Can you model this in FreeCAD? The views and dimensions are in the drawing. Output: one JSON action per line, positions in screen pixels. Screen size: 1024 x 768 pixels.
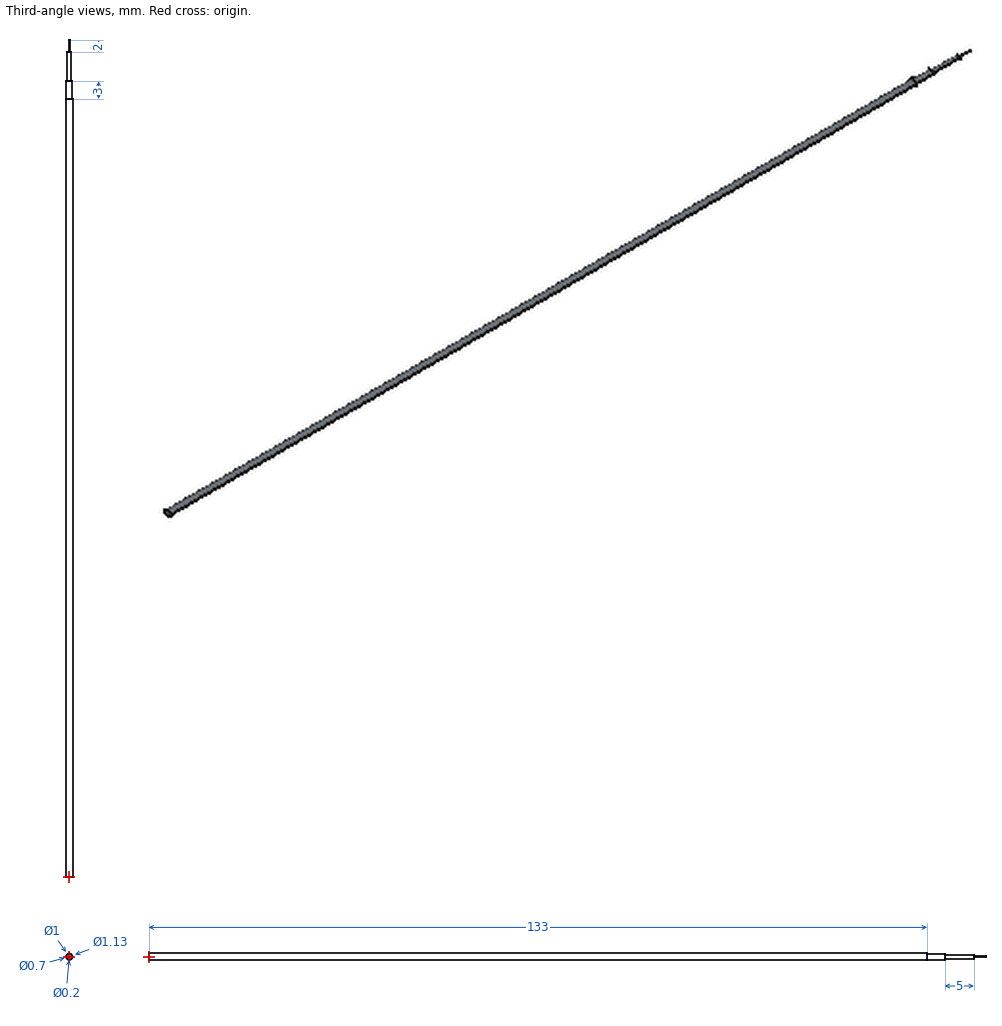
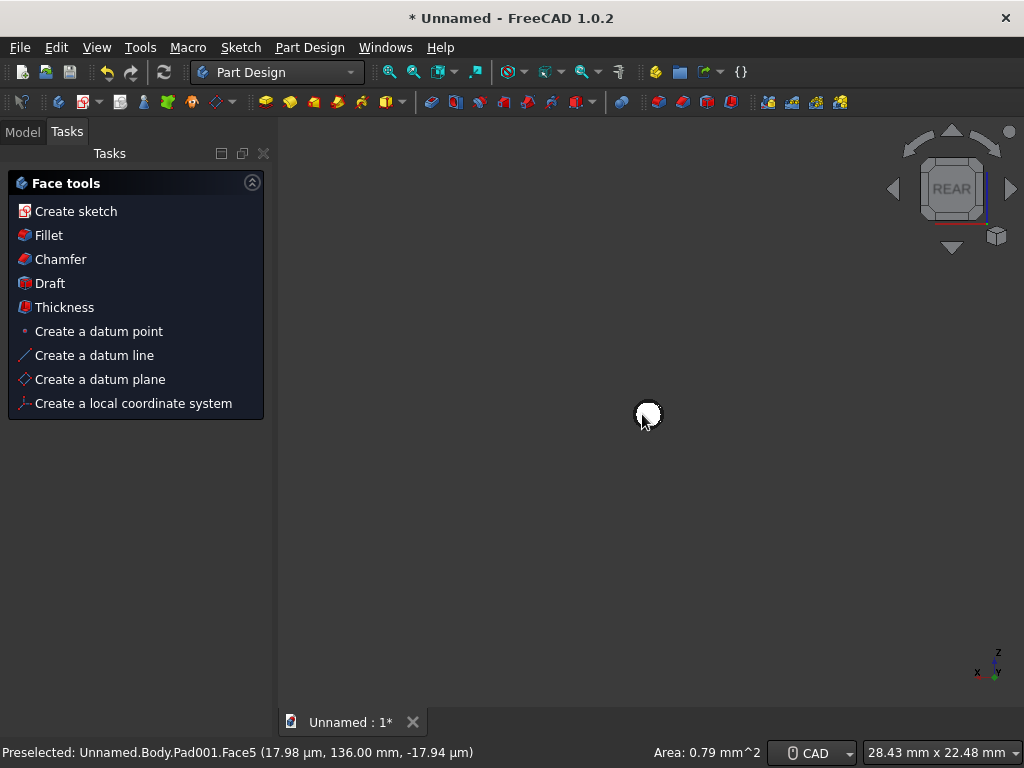
{"action": "left_click", "coordinate": [84, 102]}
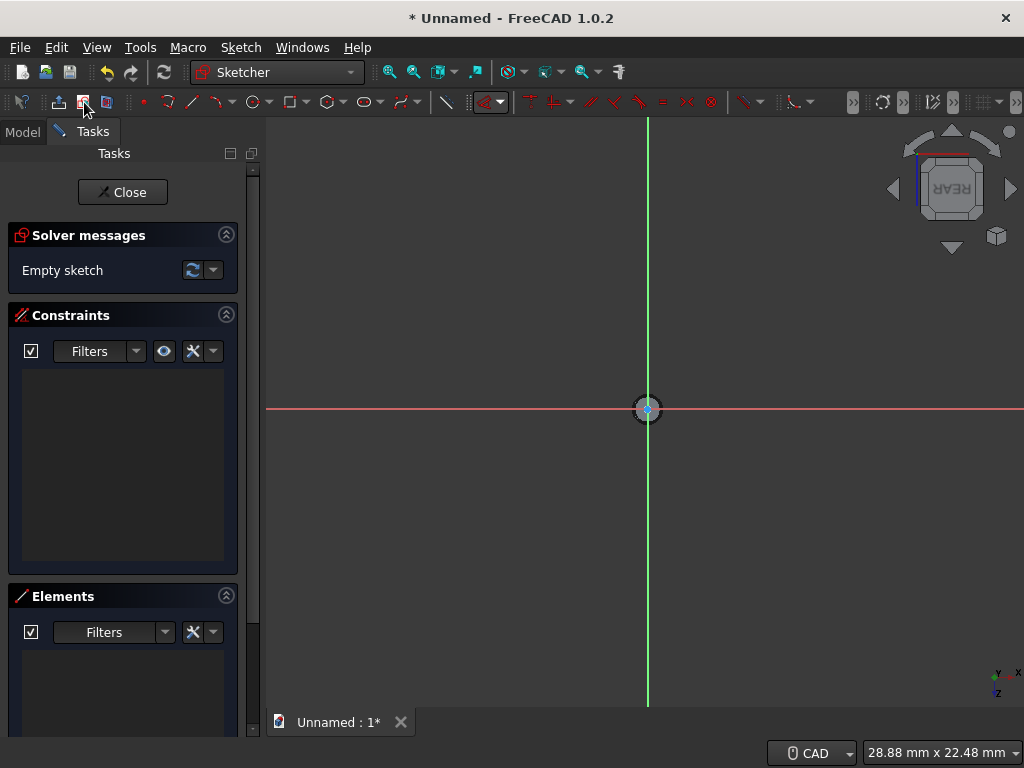
{"action": "scroll", "coordinate": [651, 409], "scroll_direction": "up", "scroll_amount": 15}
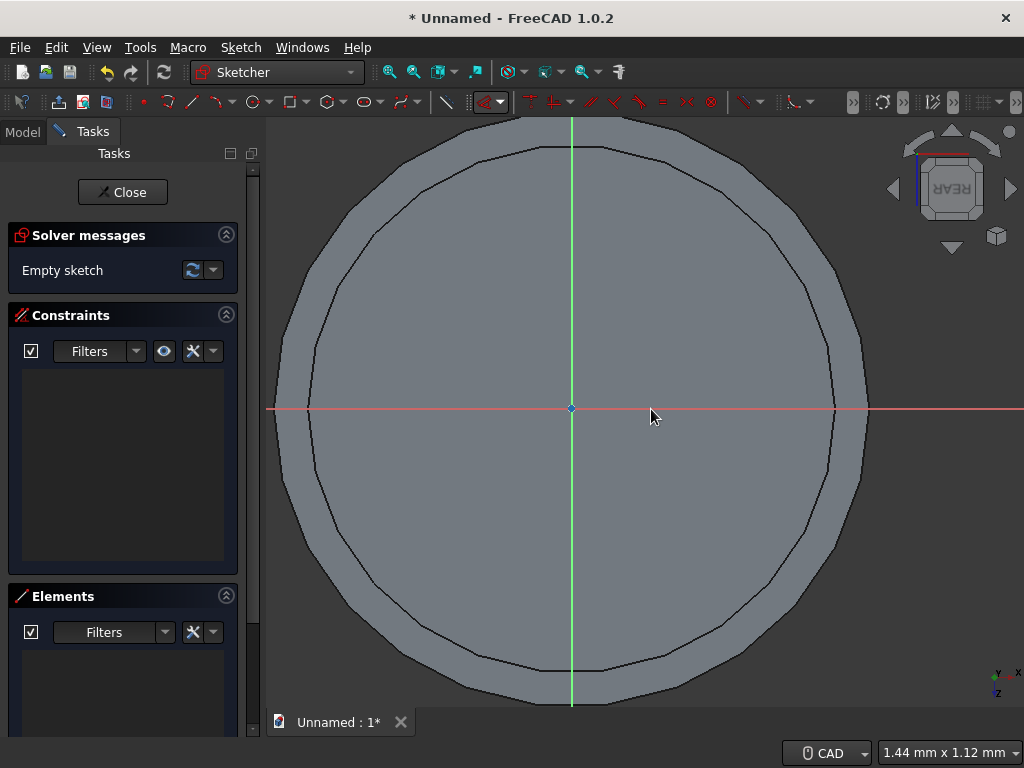
{"action": "left_click", "coordinate": [254, 102]}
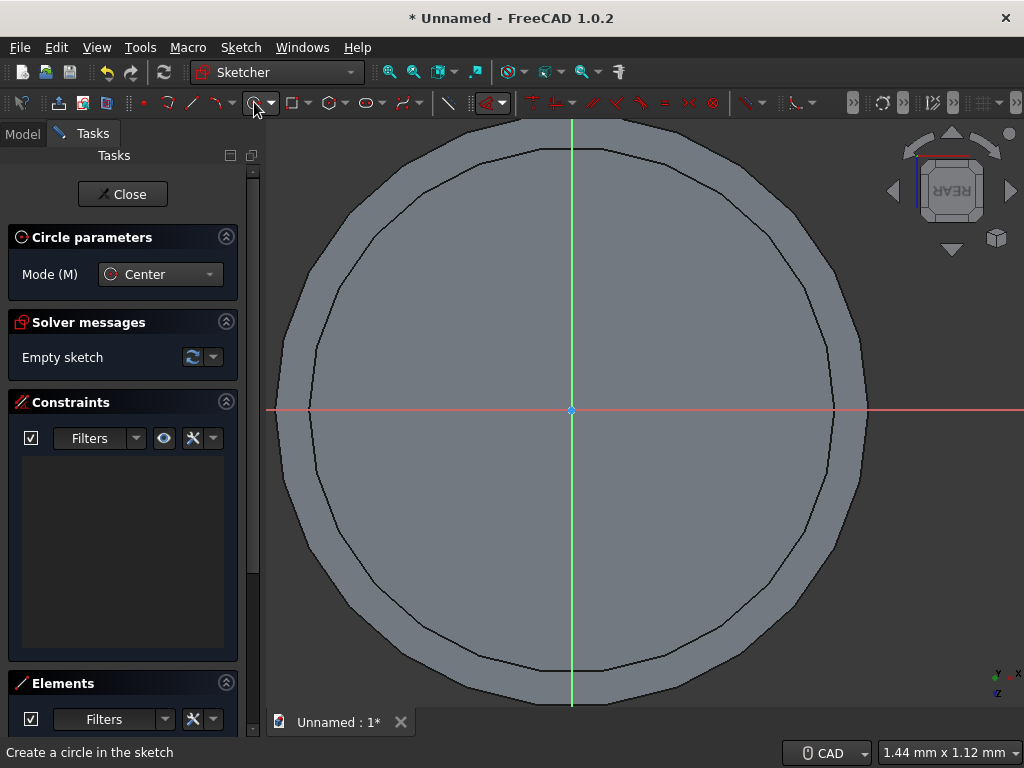
{"action": "left_click", "coordinate": [572, 410]}
{"action": "left_click", "coordinate": [702, 280]}
{"action": "key", "text": "Escape"}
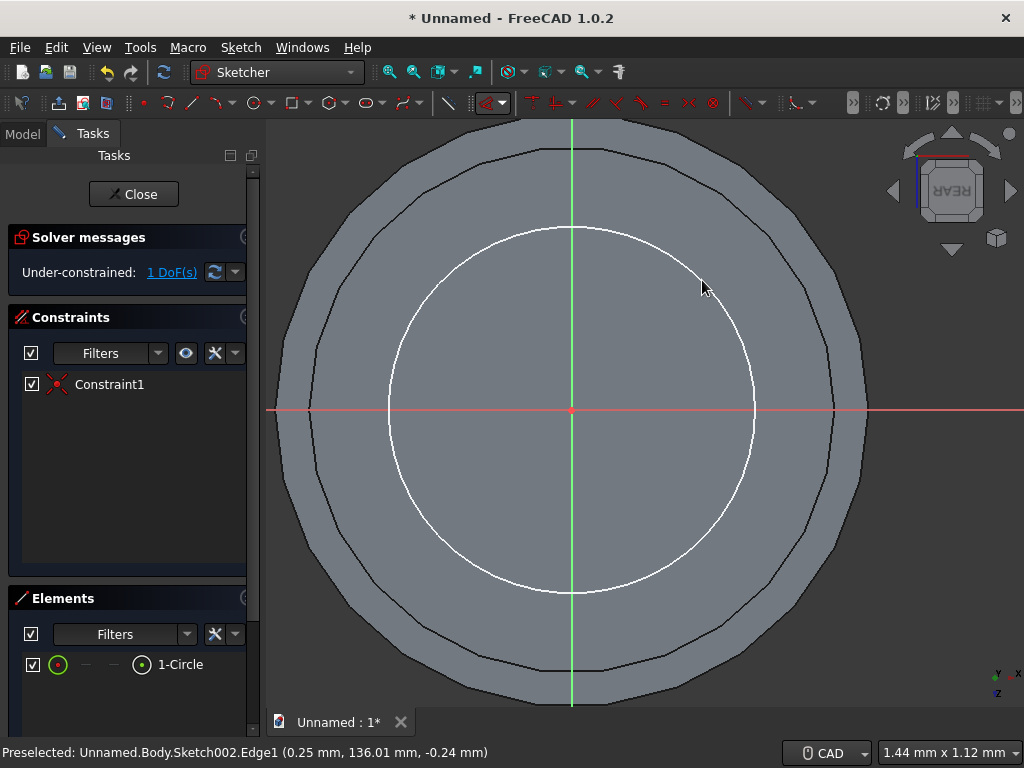
{"action": "left_click", "coordinate": [701, 280]}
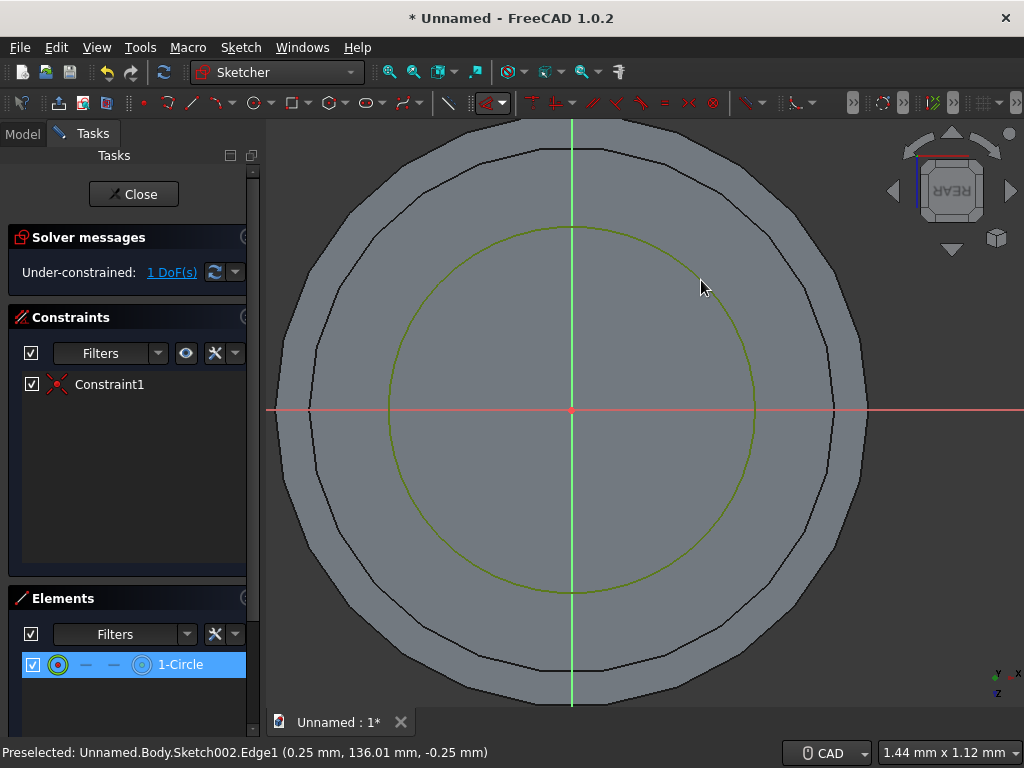
{"action": "left_click", "coordinate": [504, 104]}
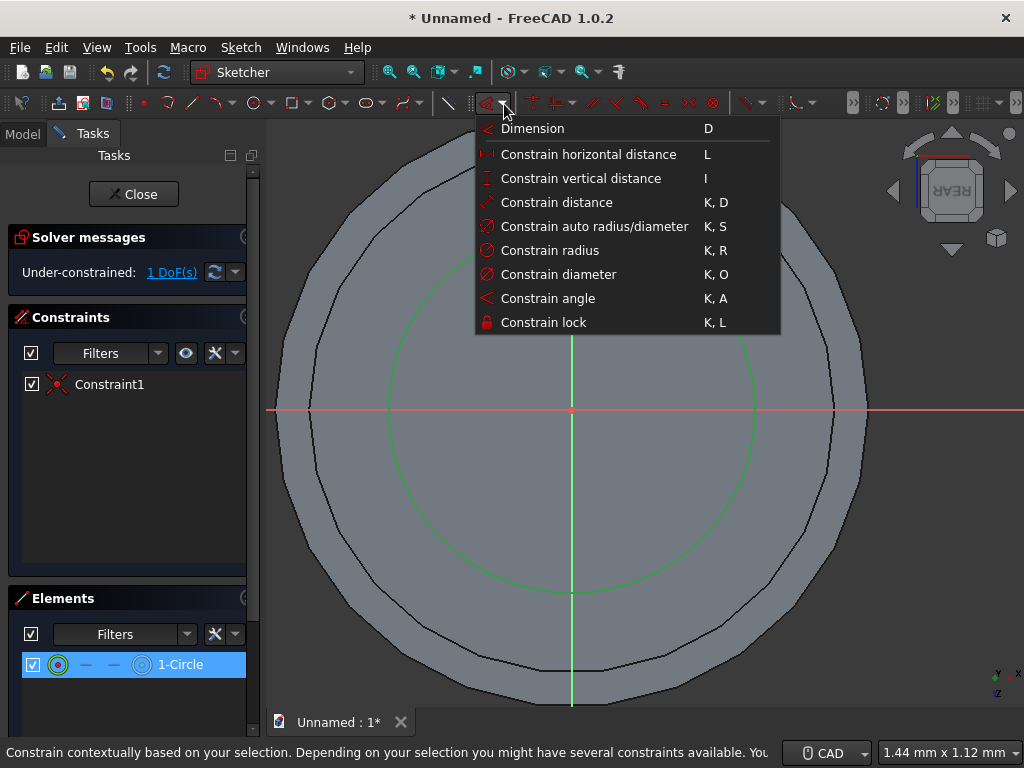
{"action": "left_click", "coordinate": [628, 274]}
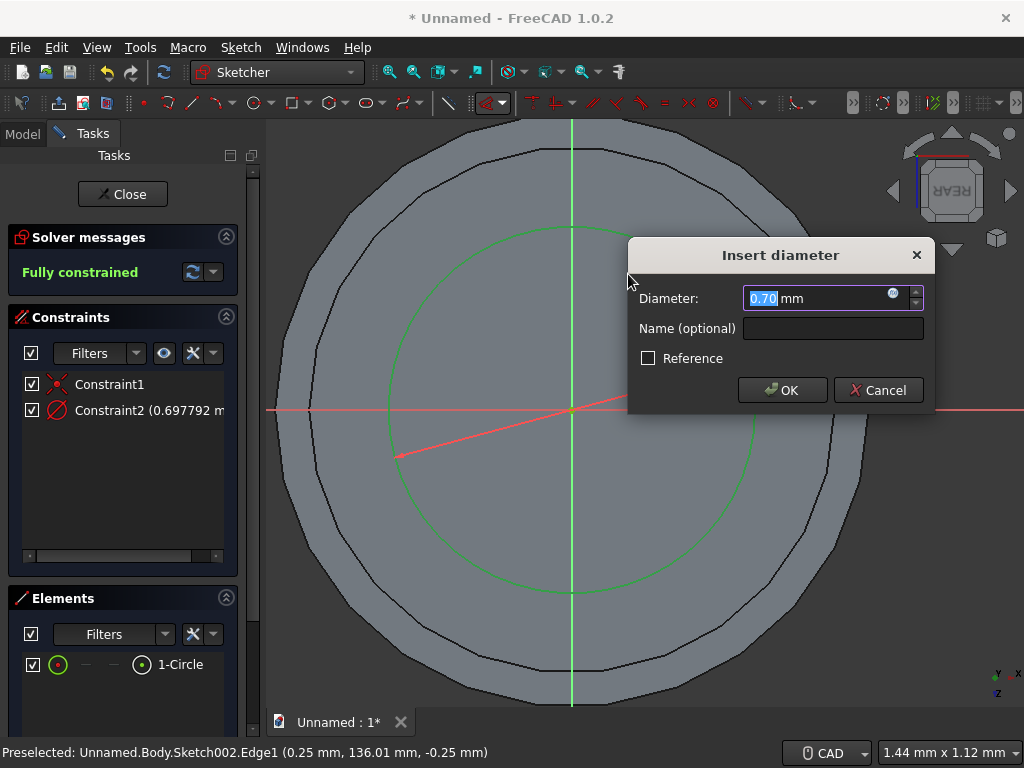
{"action": "type", "text": "0.7"}
{"action": "key", "text": "Return"}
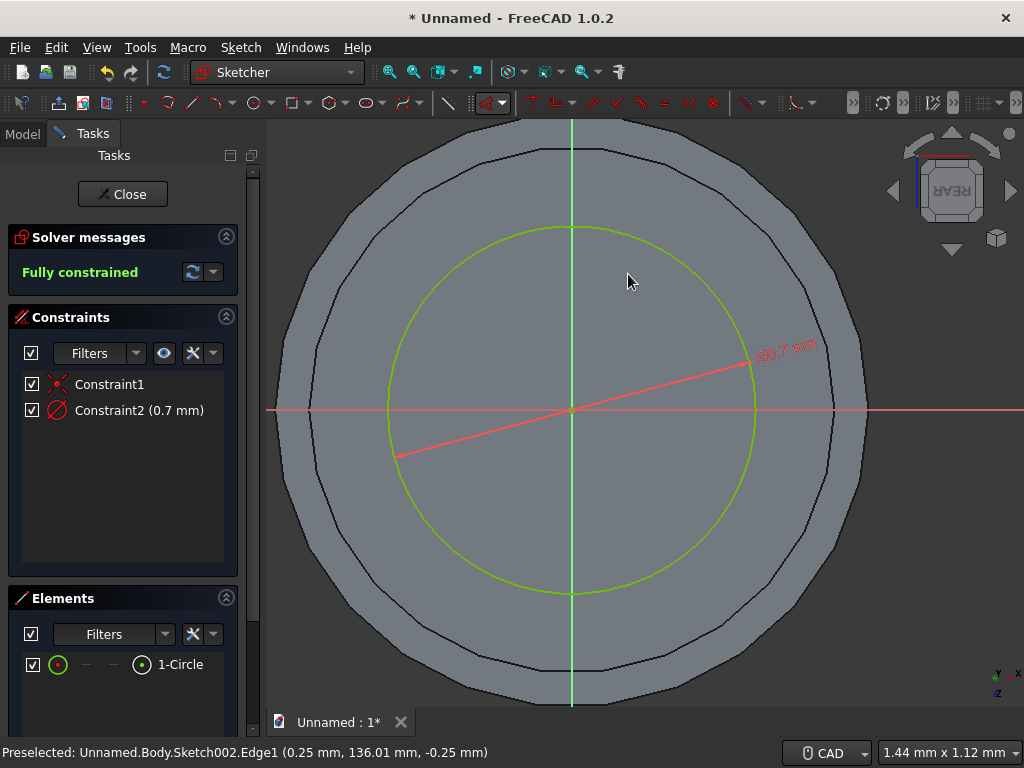
{"action": "left_click", "coordinate": [123, 194]}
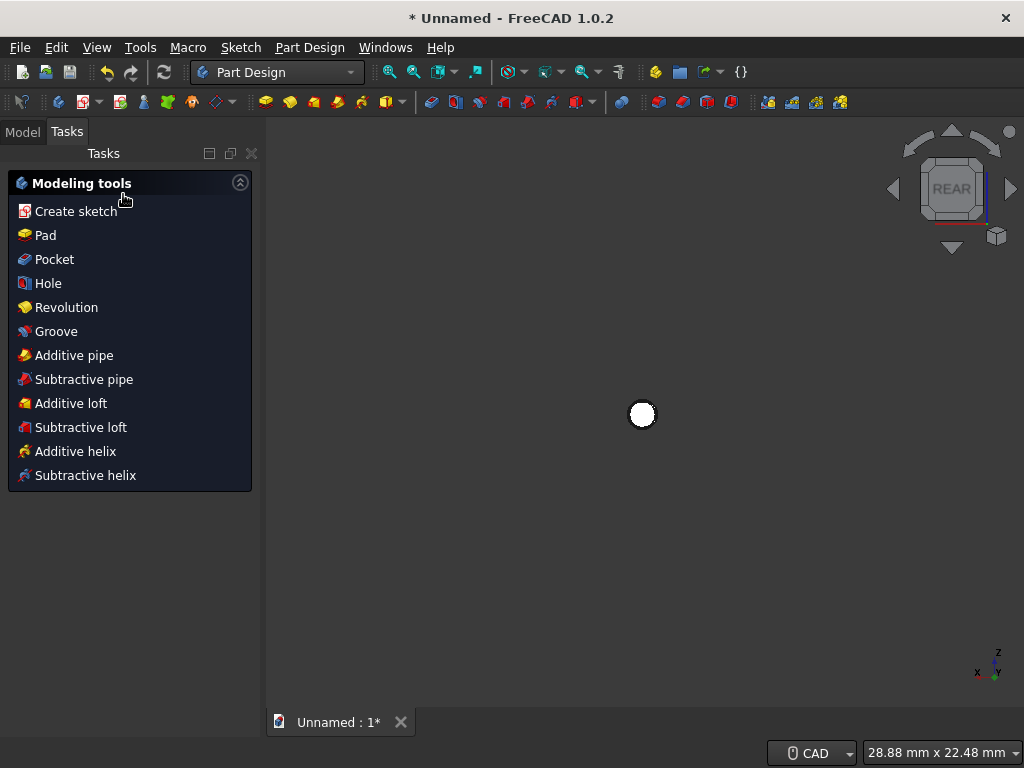
{"action": "left_click", "coordinate": [266, 102]}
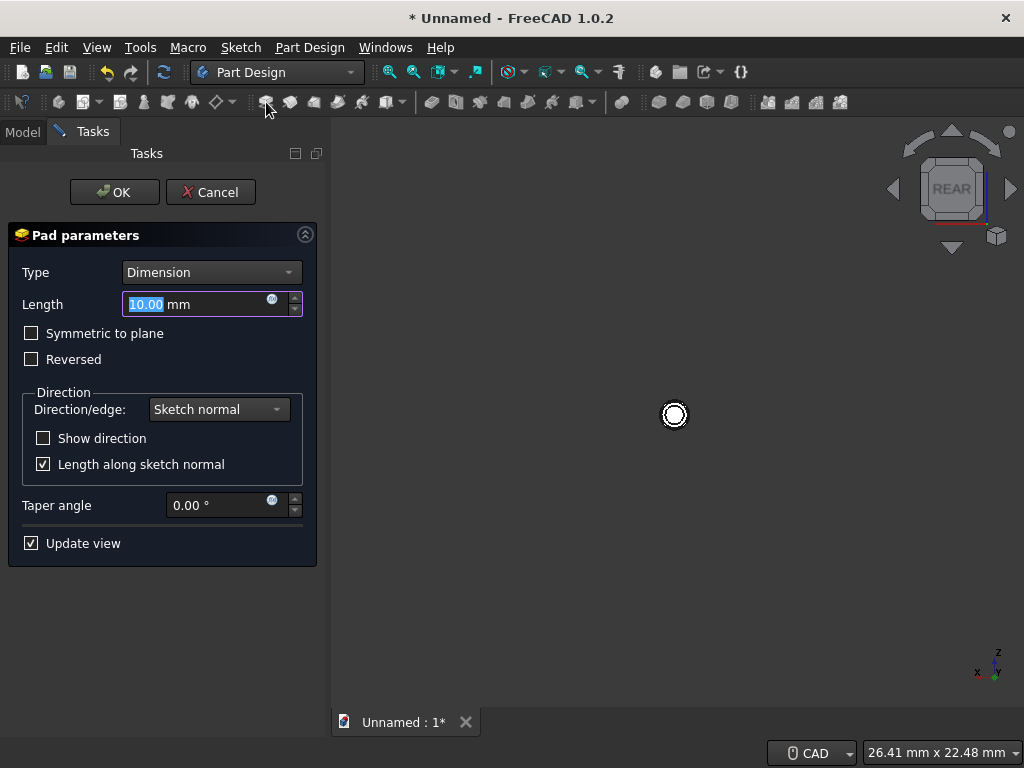
{"action": "type", "text": "5"}
{"action": "key", "text": "Tab"}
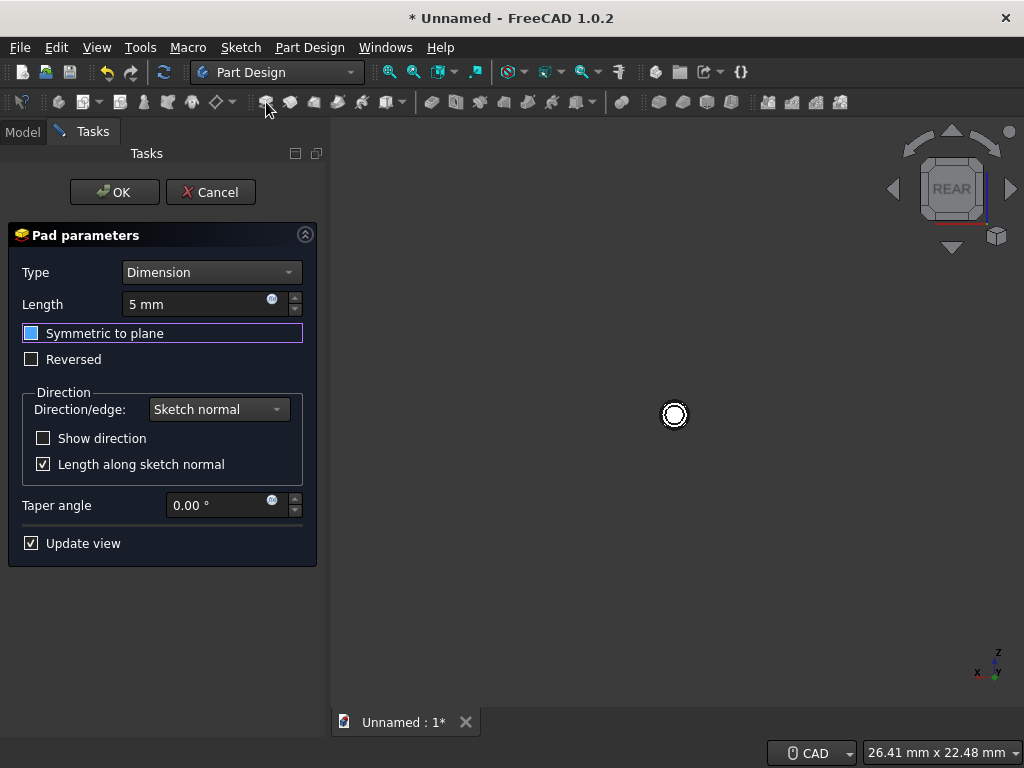
{"action": "left_click", "coordinate": [115, 192]}